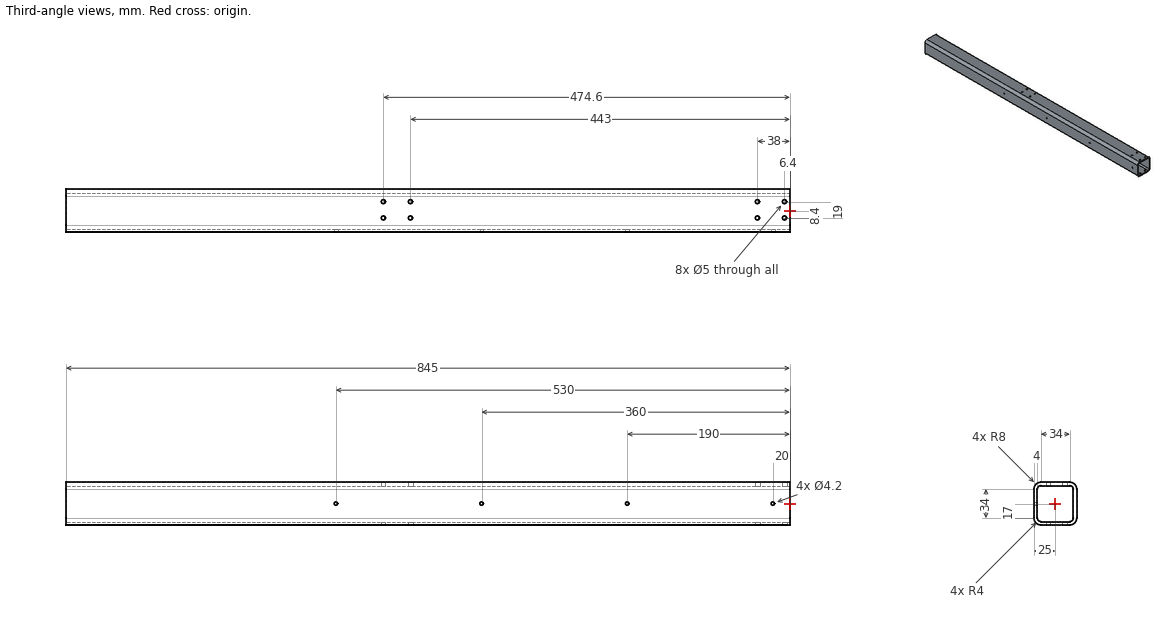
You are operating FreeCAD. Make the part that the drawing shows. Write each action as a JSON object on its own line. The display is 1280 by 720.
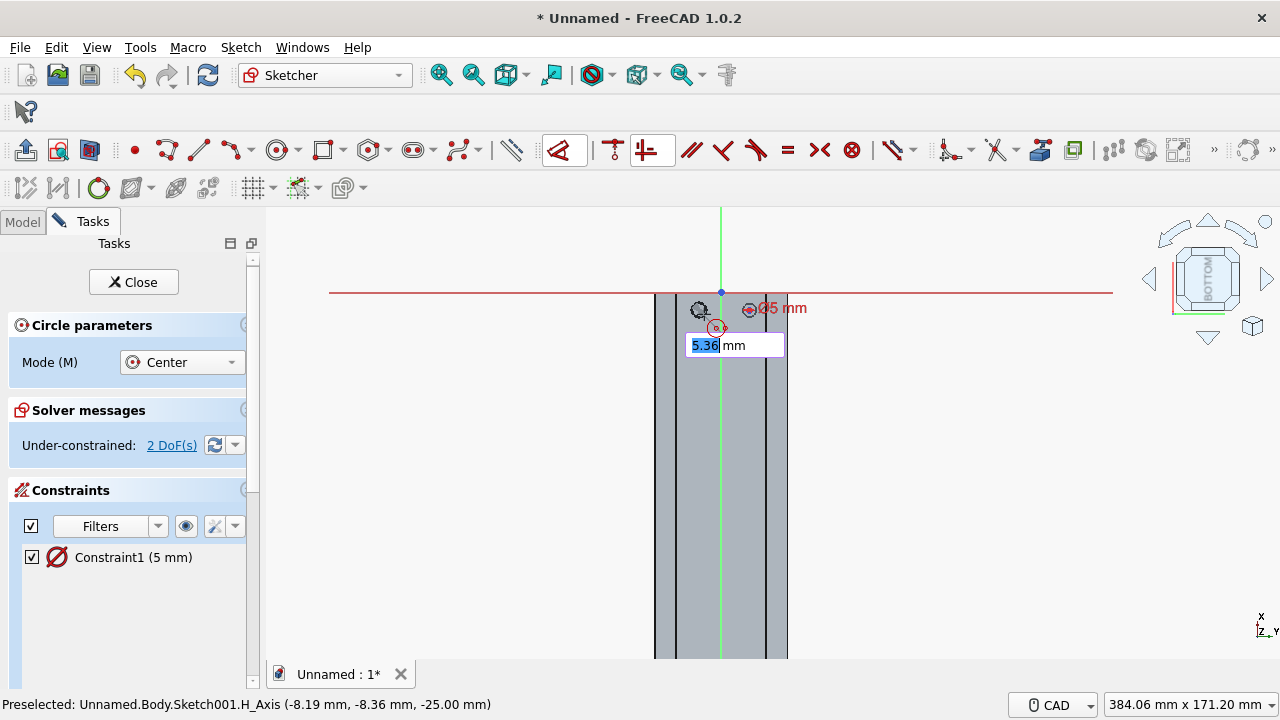
{"action": "type", "text": "5"}
{"action": "key", "text": "Return"}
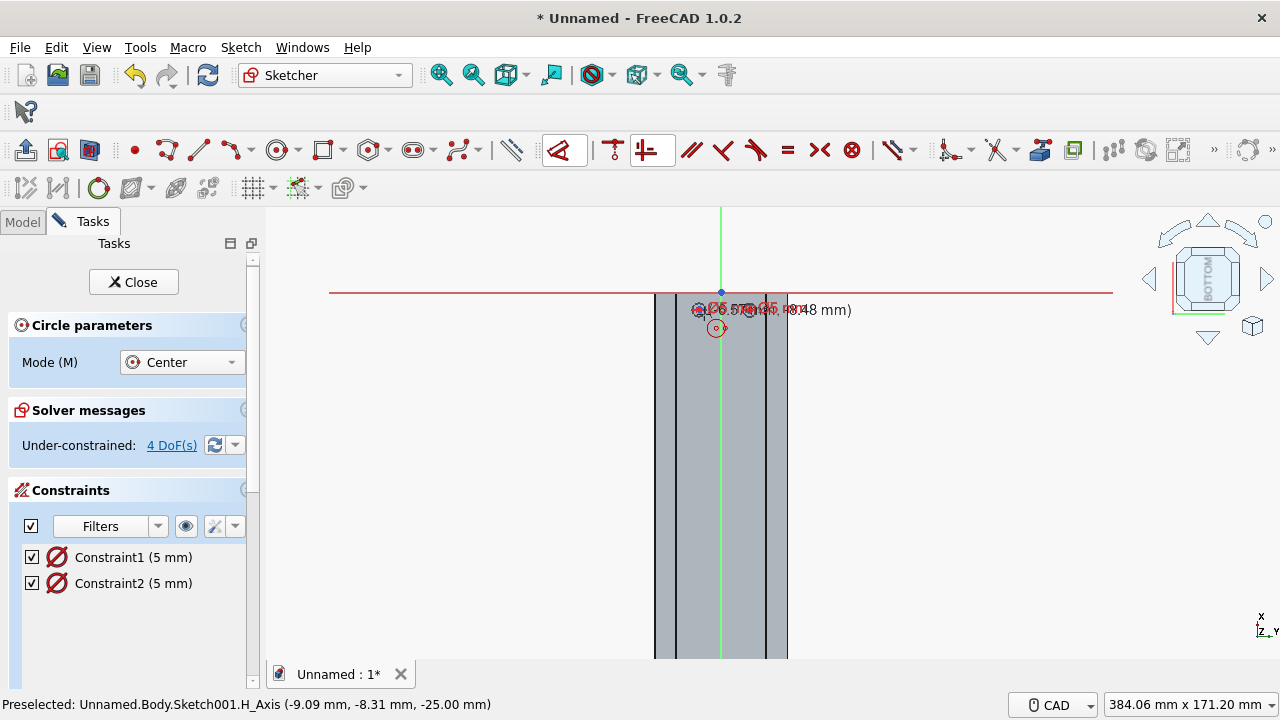
{"action": "scroll", "coordinate": [749, 393], "scroll_direction": "up", "scroll_amount": 7}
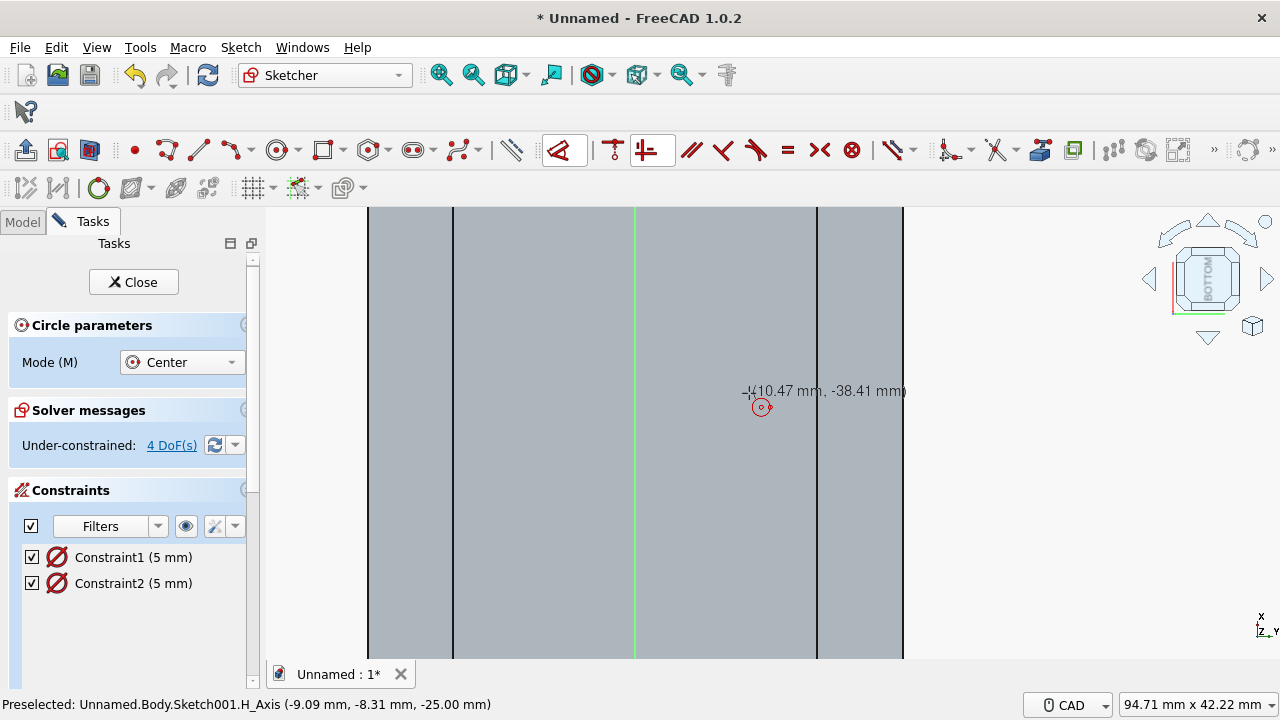
{"action": "scroll", "coordinate": [708, 323], "scroll_direction": "down", "scroll_amount": 15}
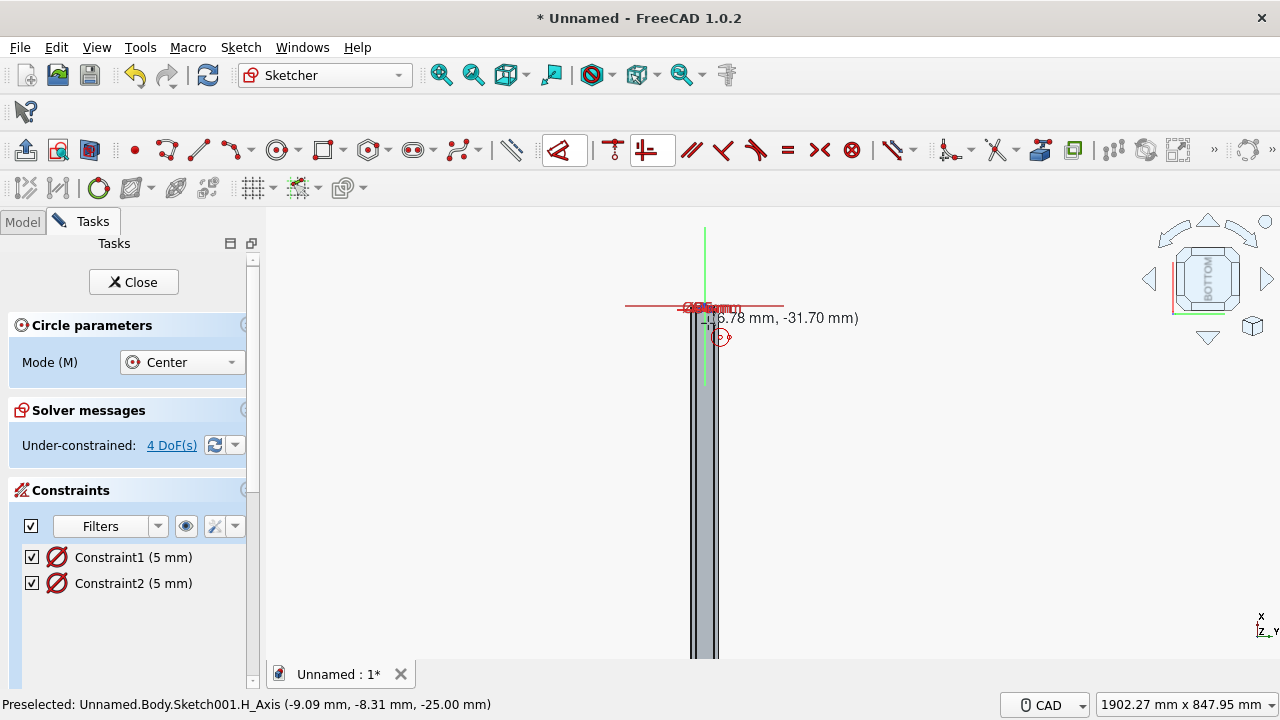
{"action": "scroll", "coordinate": [710, 327], "scroll_direction": "up", "scroll_amount": 6}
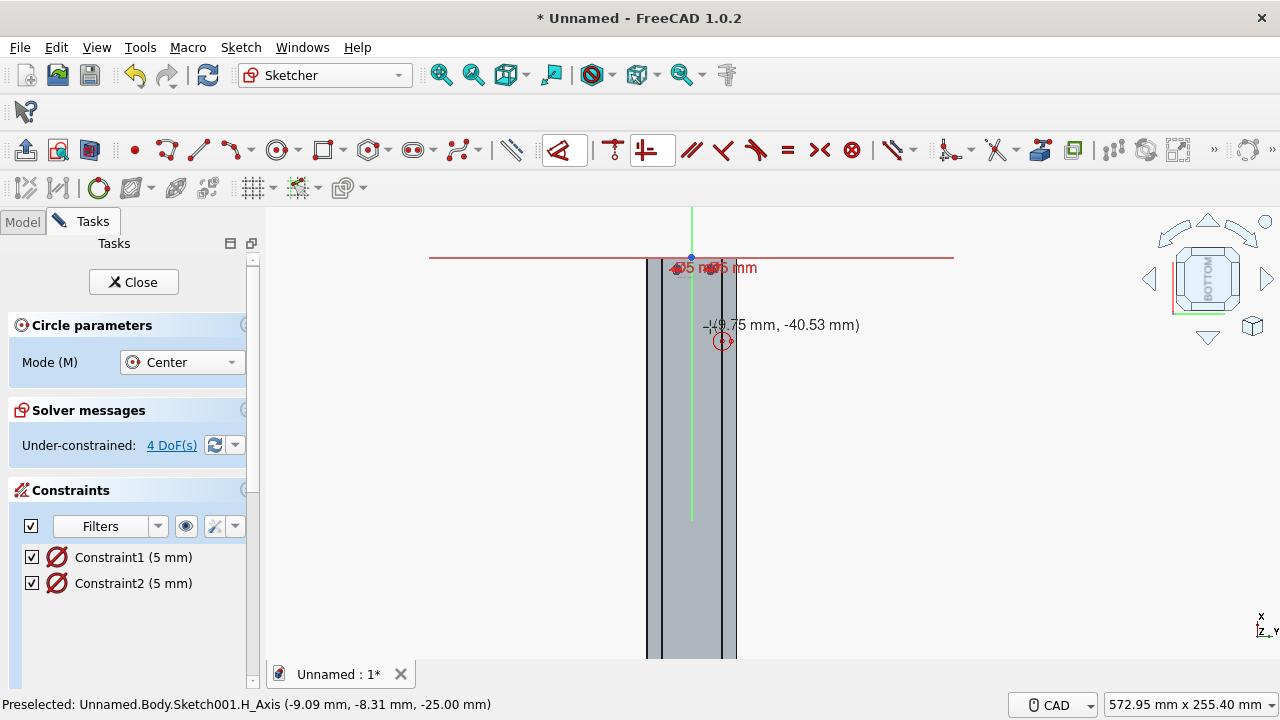
{"action": "left_click", "coordinate": [710, 325]}
{"action": "mouse_move", "coordinate": [714, 322]}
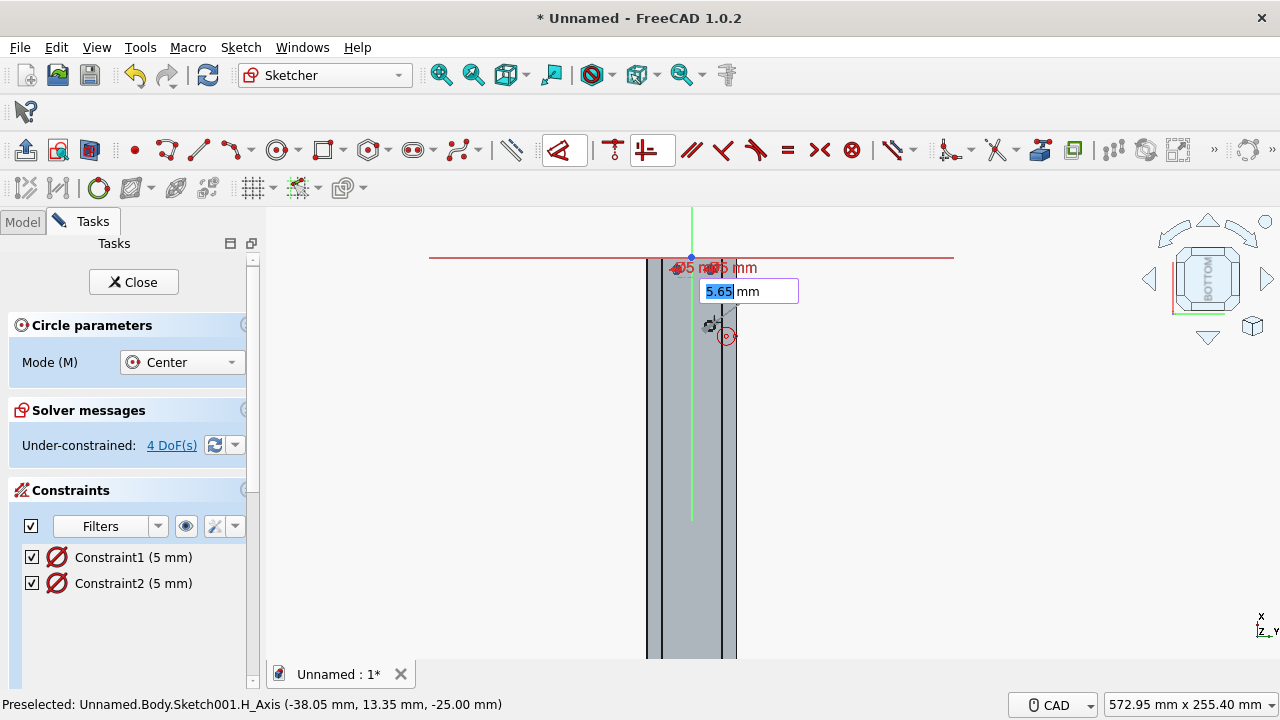
{"action": "type", "text": "5"}
{"action": "key", "text": "Return"}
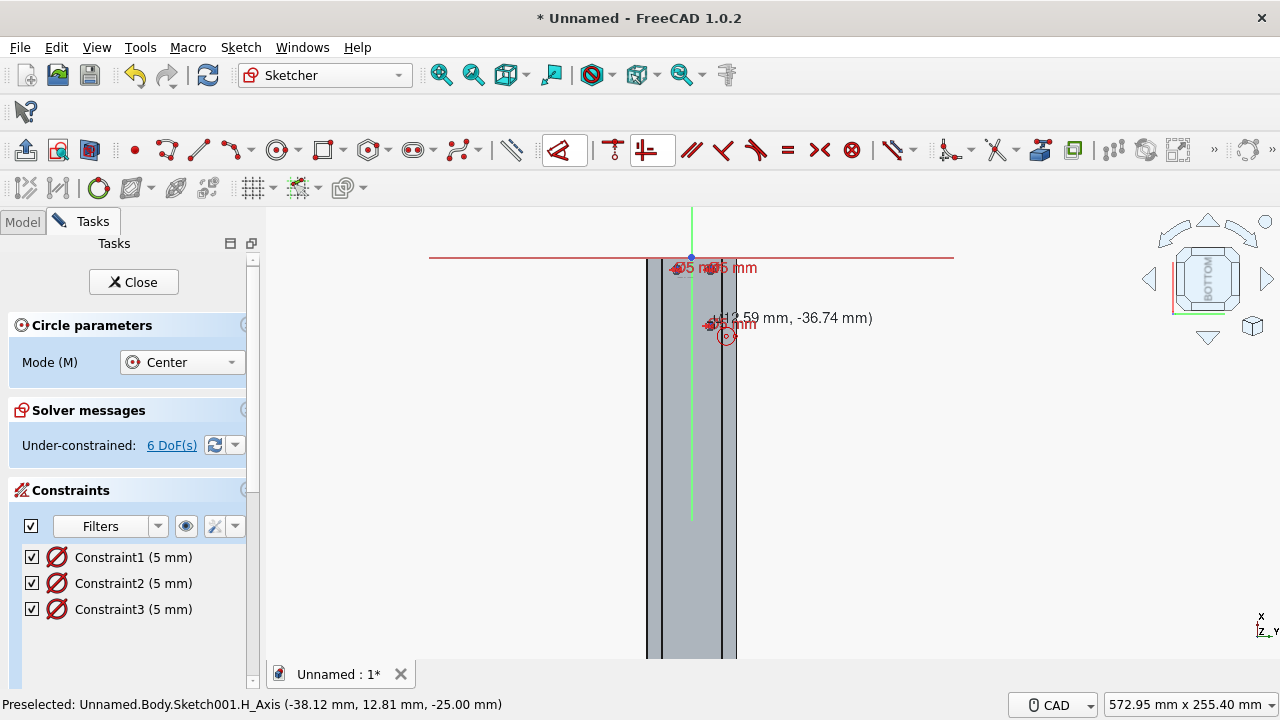
{"action": "scroll", "coordinate": [677, 325], "scroll_direction": "up", "scroll_amount": 9}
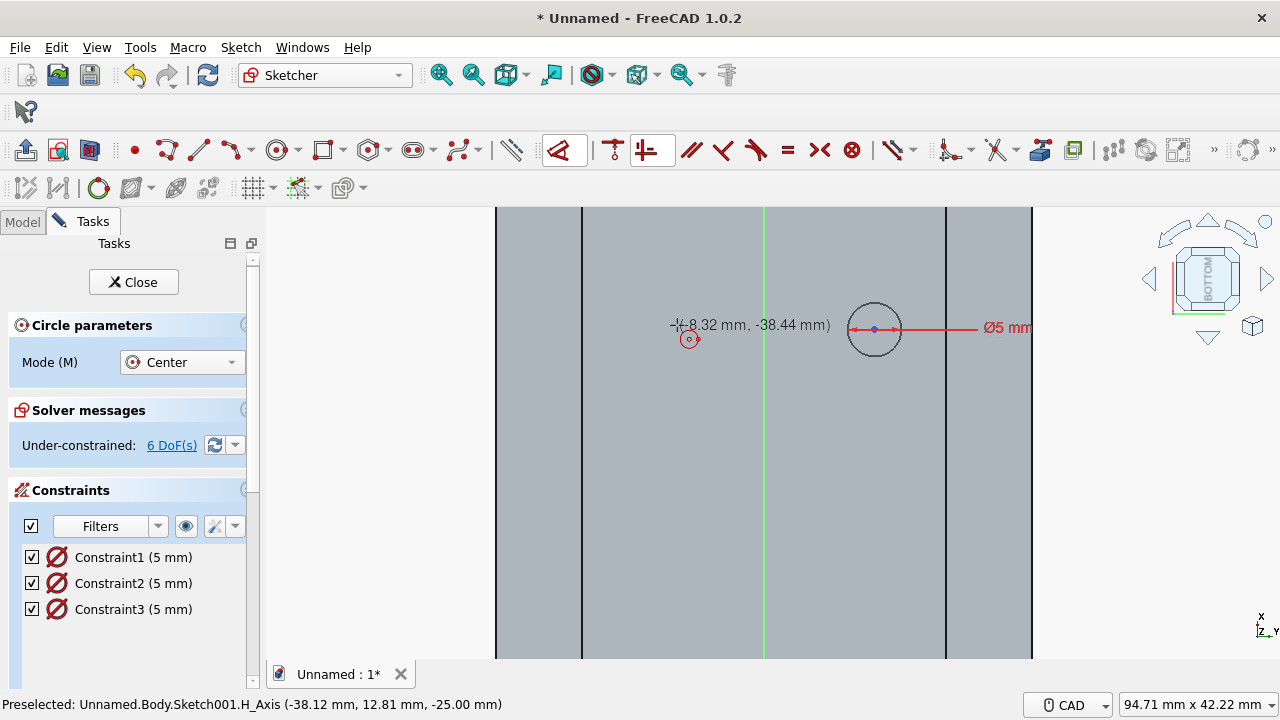
{"action": "scroll", "coordinate": [701, 326], "scroll_direction": "down", "scroll_amount": 15}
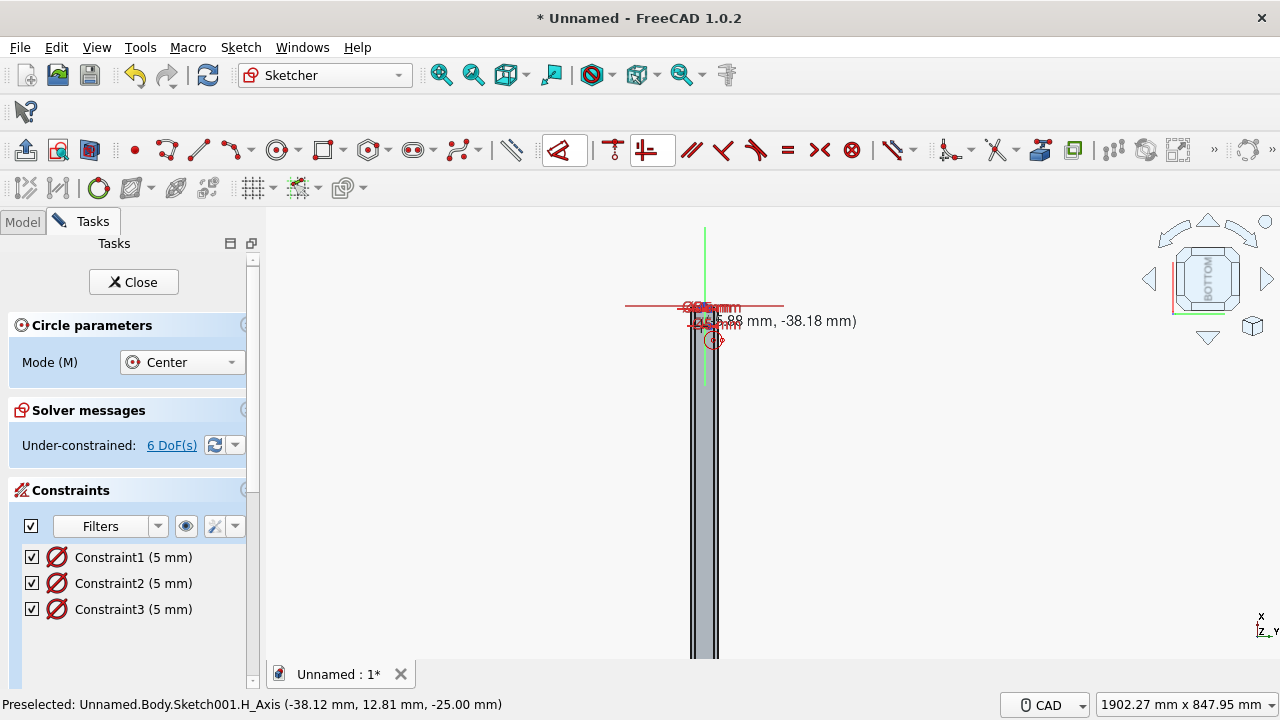
{"action": "scroll", "coordinate": [700, 326], "scroll_direction": "up", "scroll_amount": 7}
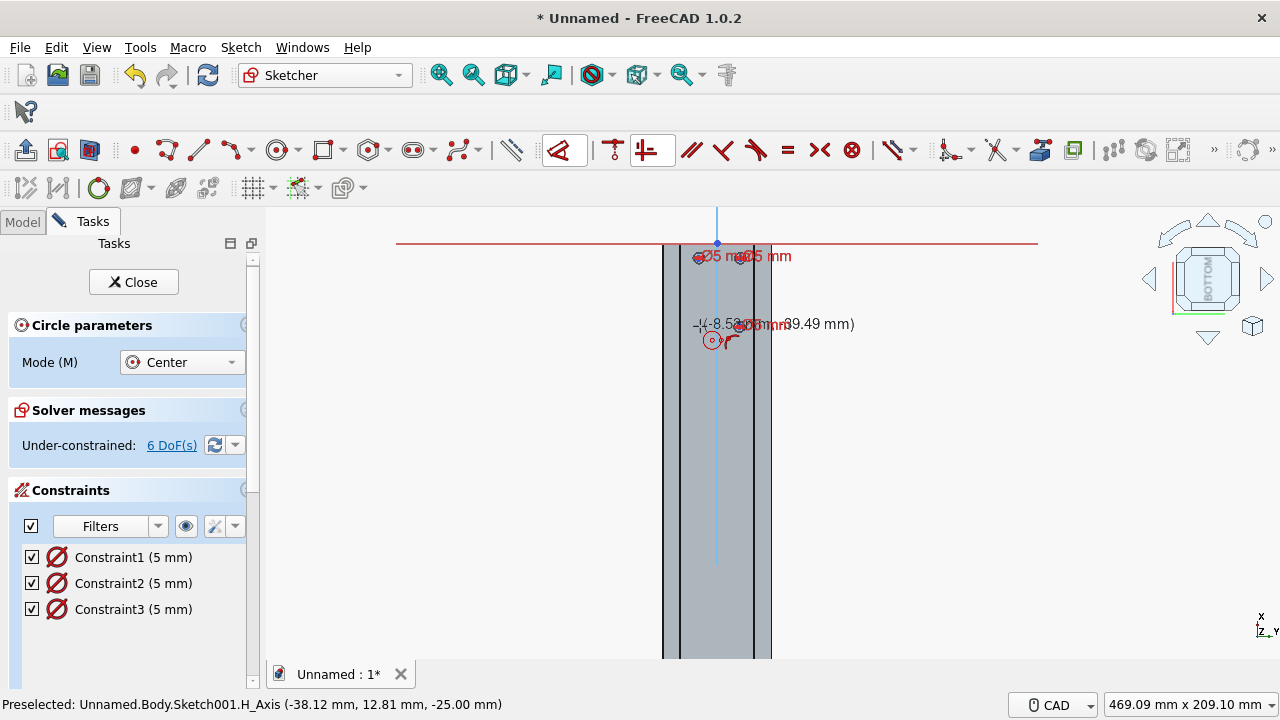
{"action": "left_click", "coordinate": [699, 326]}
{"action": "mouse_move", "coordinate": [703, 322]}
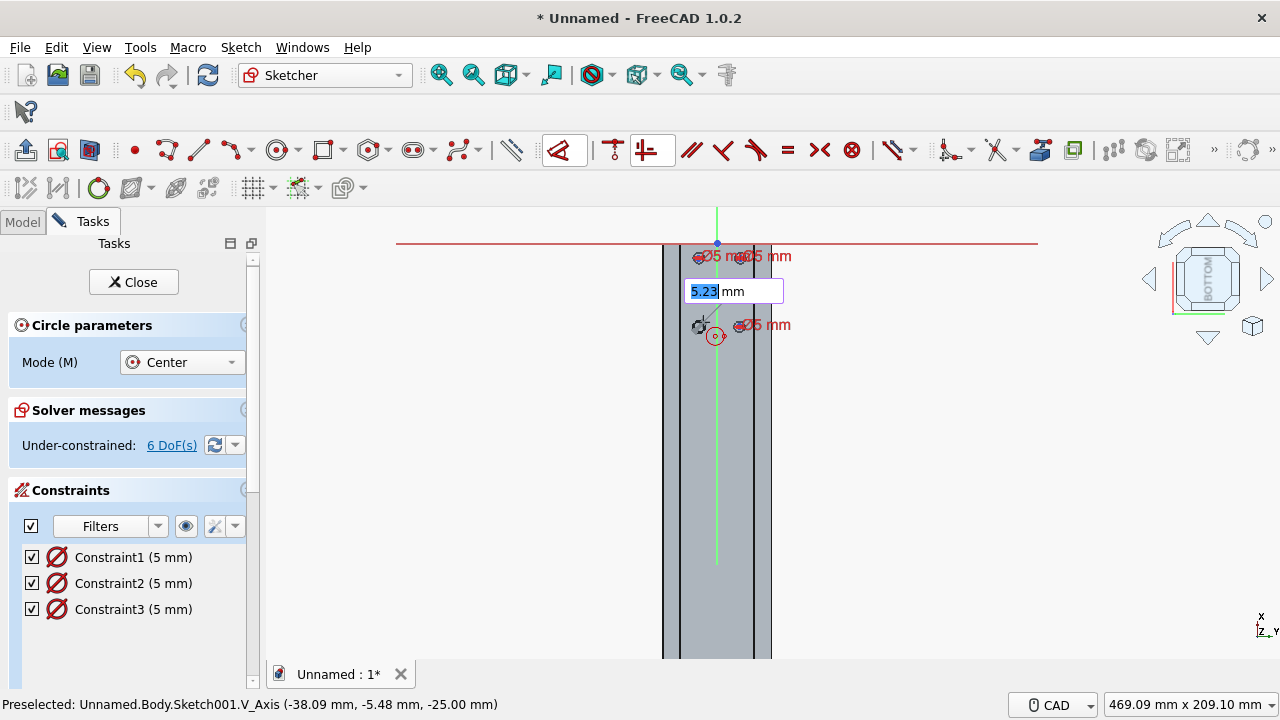
{"action": "type", "text": "5"}
{"action": "key", "text": "Return"}